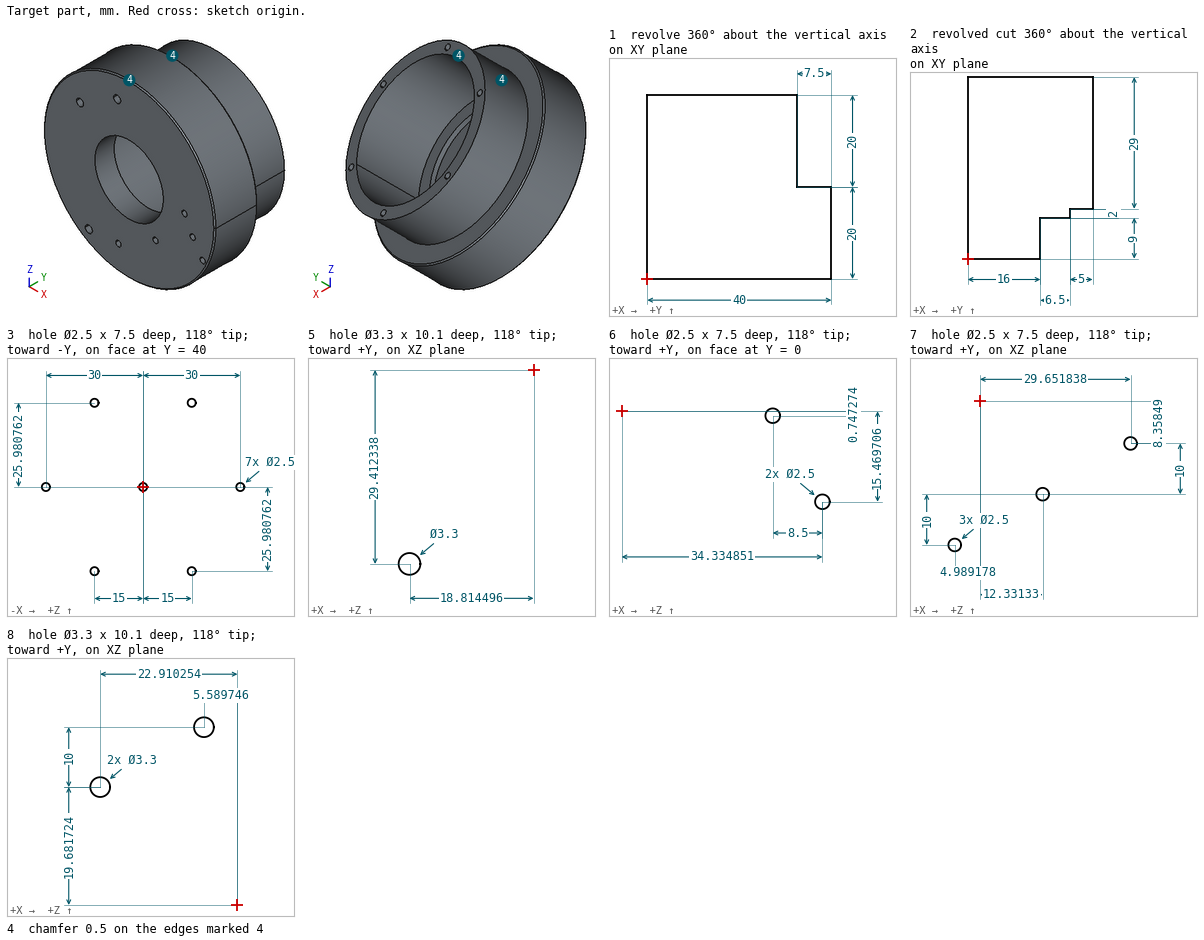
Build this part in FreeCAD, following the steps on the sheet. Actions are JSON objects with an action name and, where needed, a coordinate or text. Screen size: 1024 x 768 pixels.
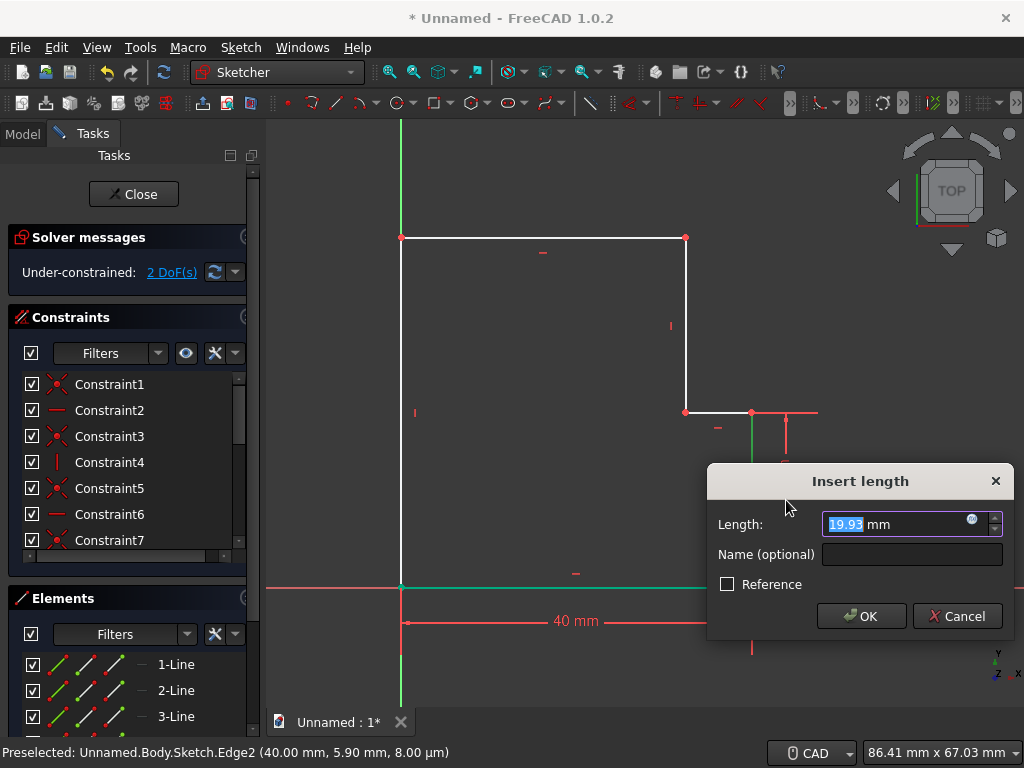
{"action": "type", "text": "20"}
{"action": "key", "text": "Return"}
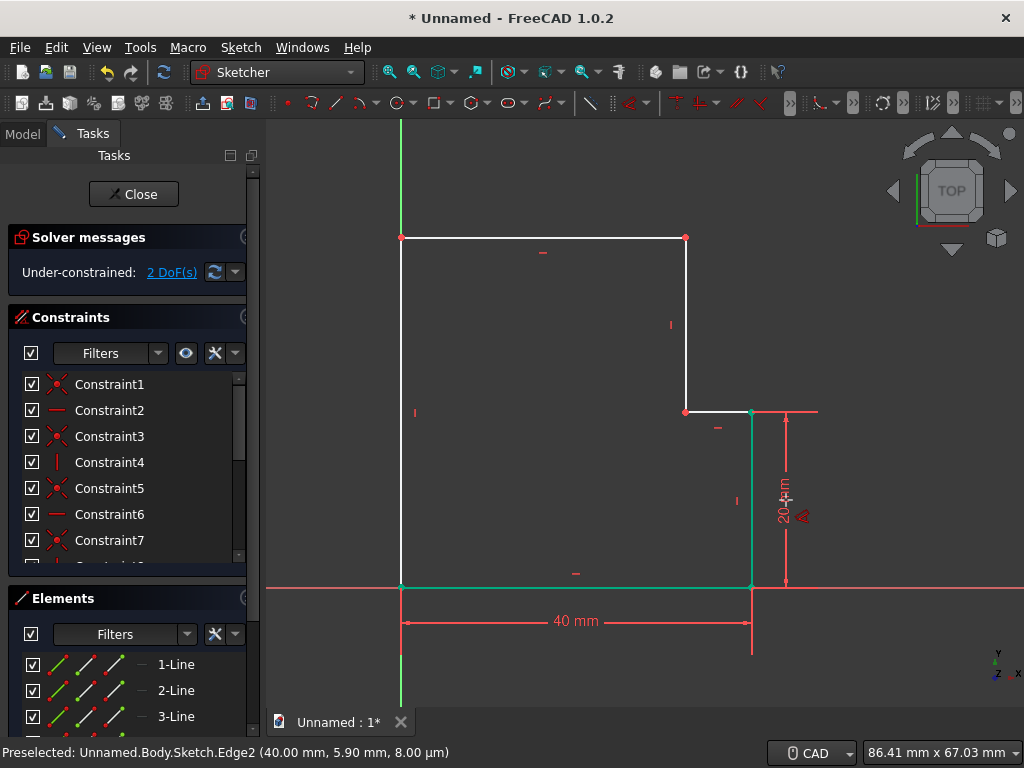
{"action": "left_click", "coordinate": [686, 360]}
{"action": "left_click", "coordinate": [720, 325]}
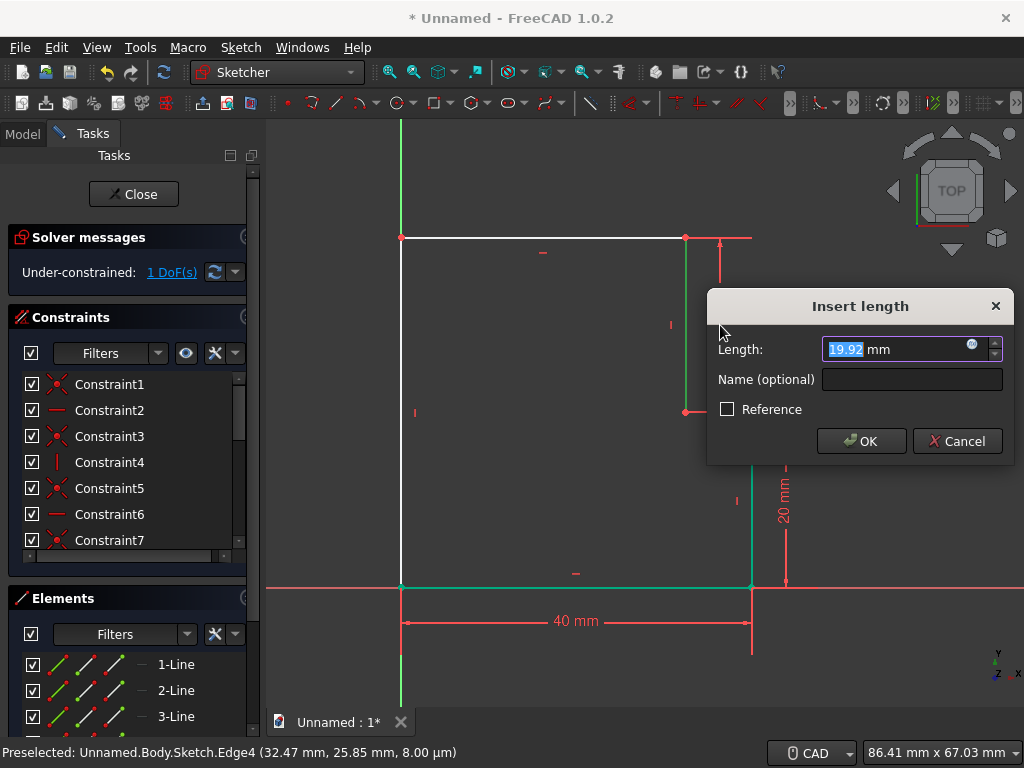
{"action": "type", "text": "20"}
{"action": "key", "text": "Return"}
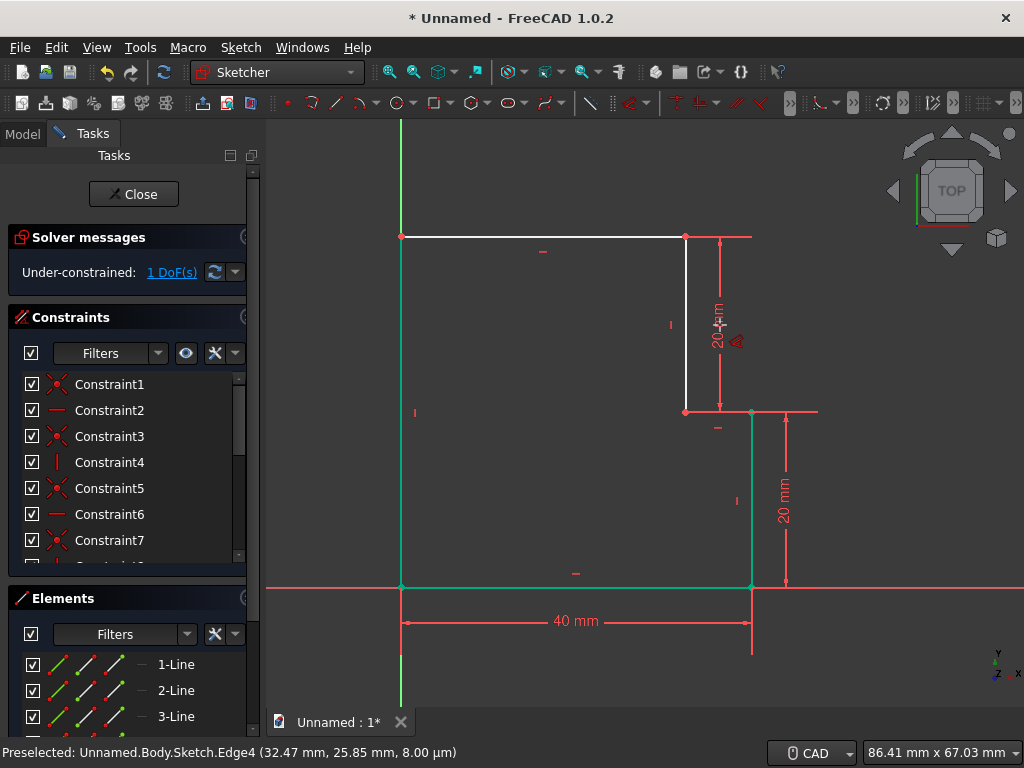
{"action": "left_click", "coordinate": [732, 412]}
{"action": "left_click", "coordinate": [719, 446]}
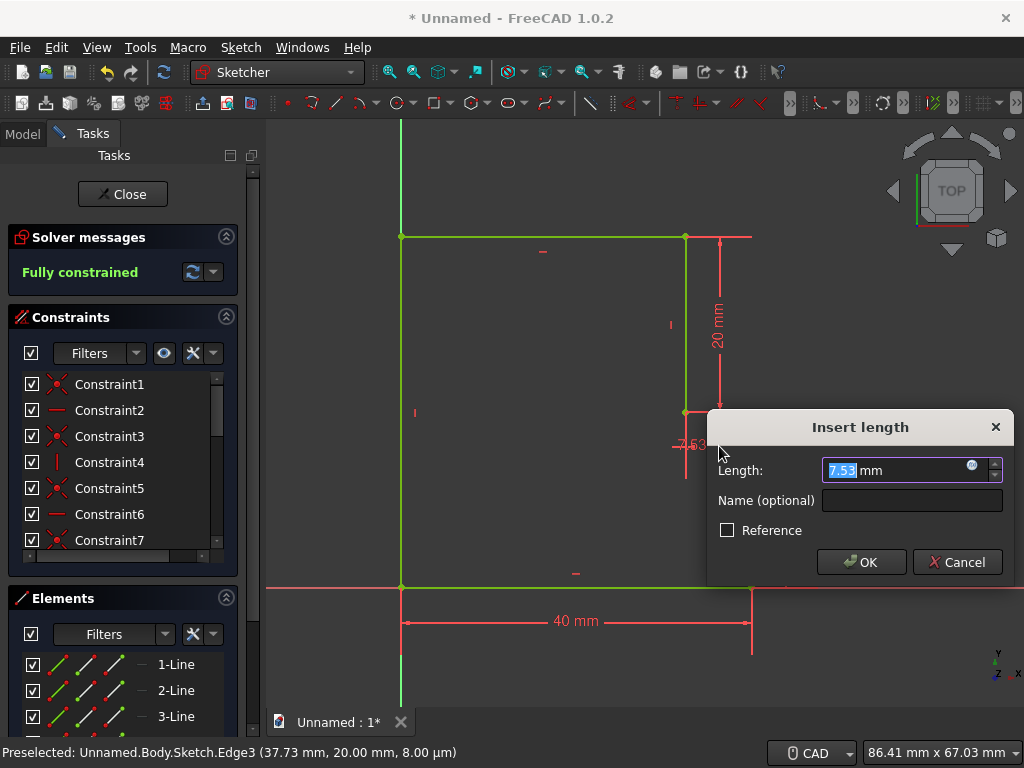
{"action": "type", "text": "7.5"}
{"action": "key", "text": "Return"}
{"action": "key", "text": "Escape"}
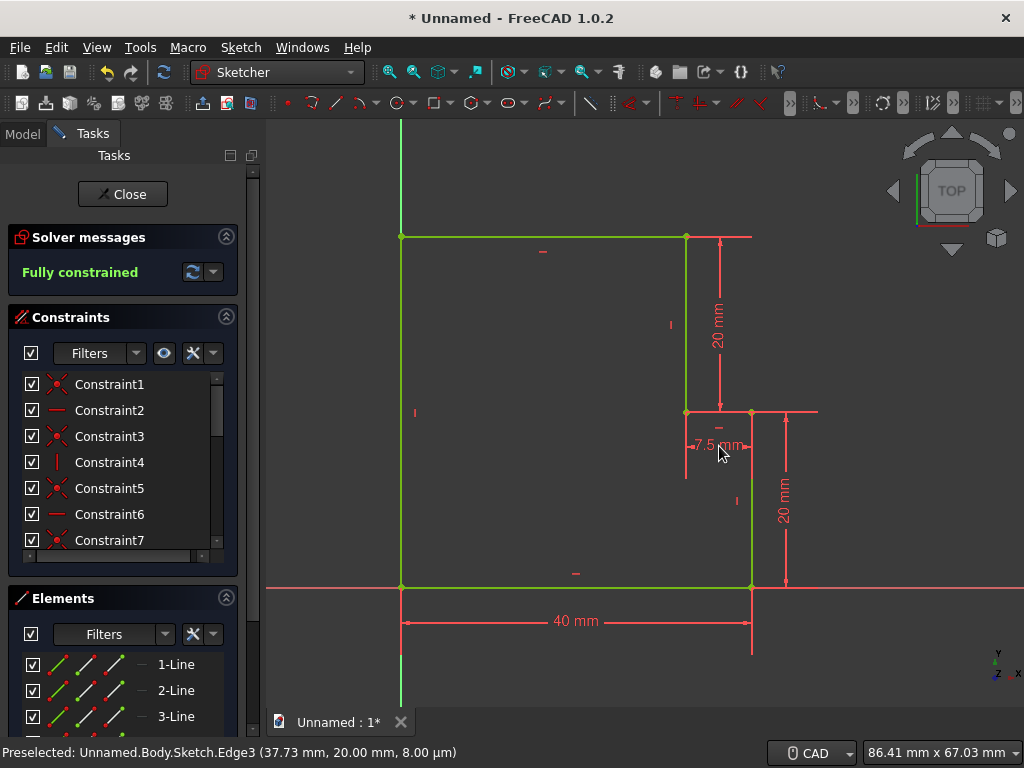
{"action": "left_click", "coordinate": [123, 194]}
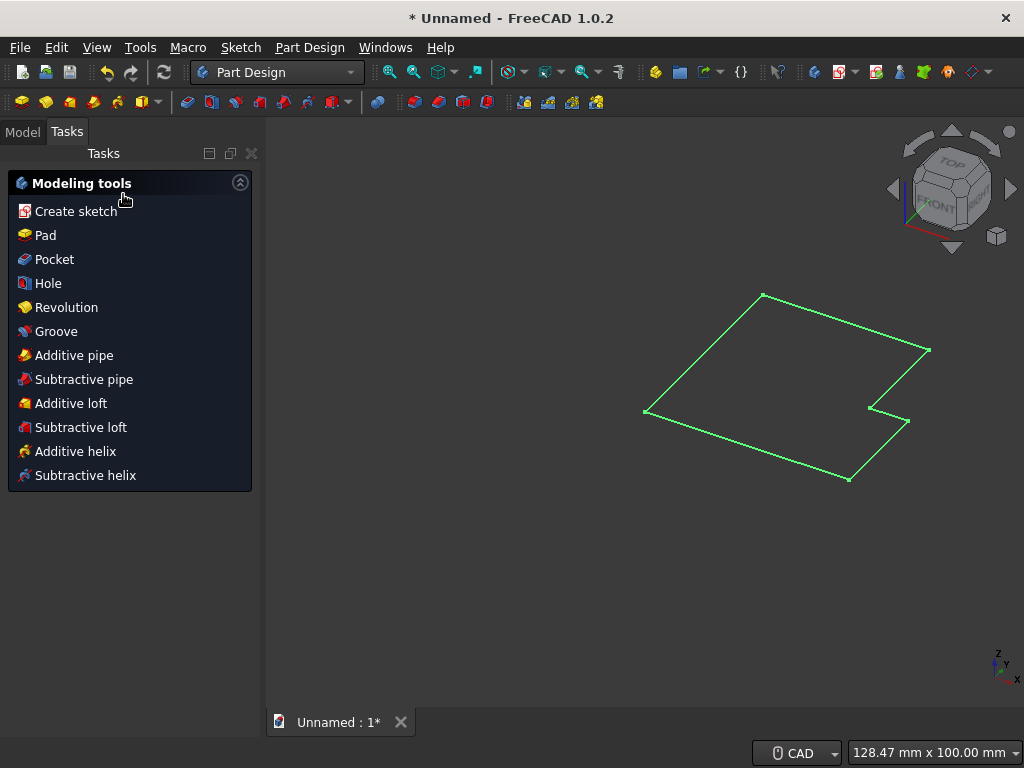
{"action": "left_click", "coordinate": [46, 102]}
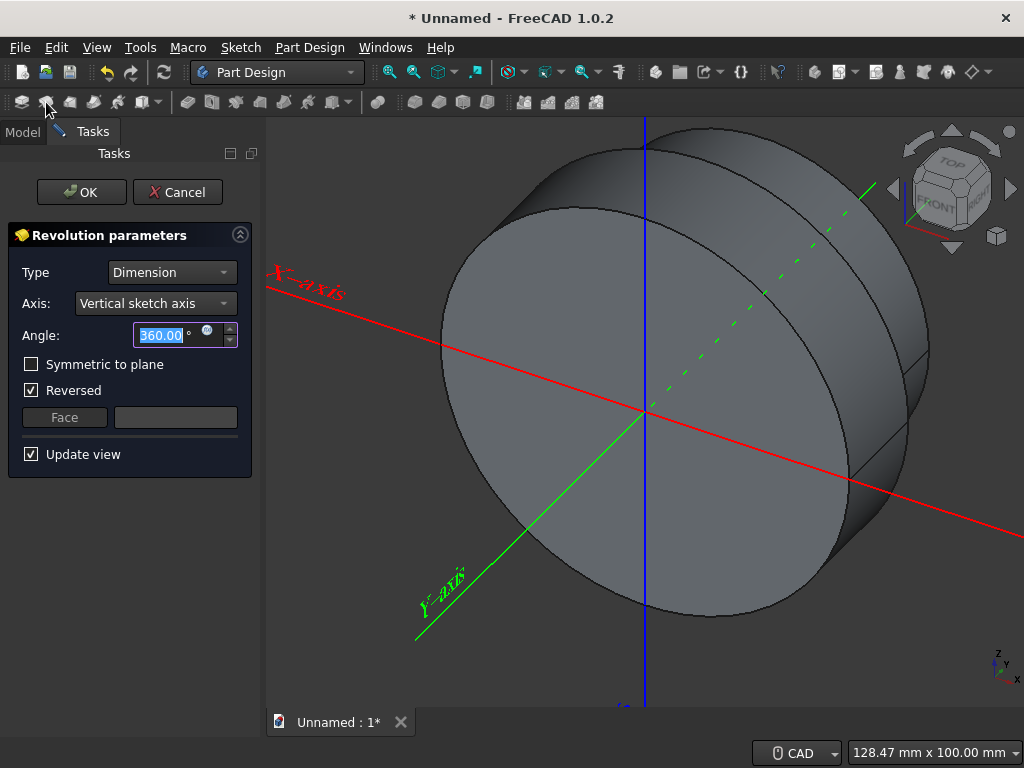
{"action": "left_click", "coordinate": [82, 192]}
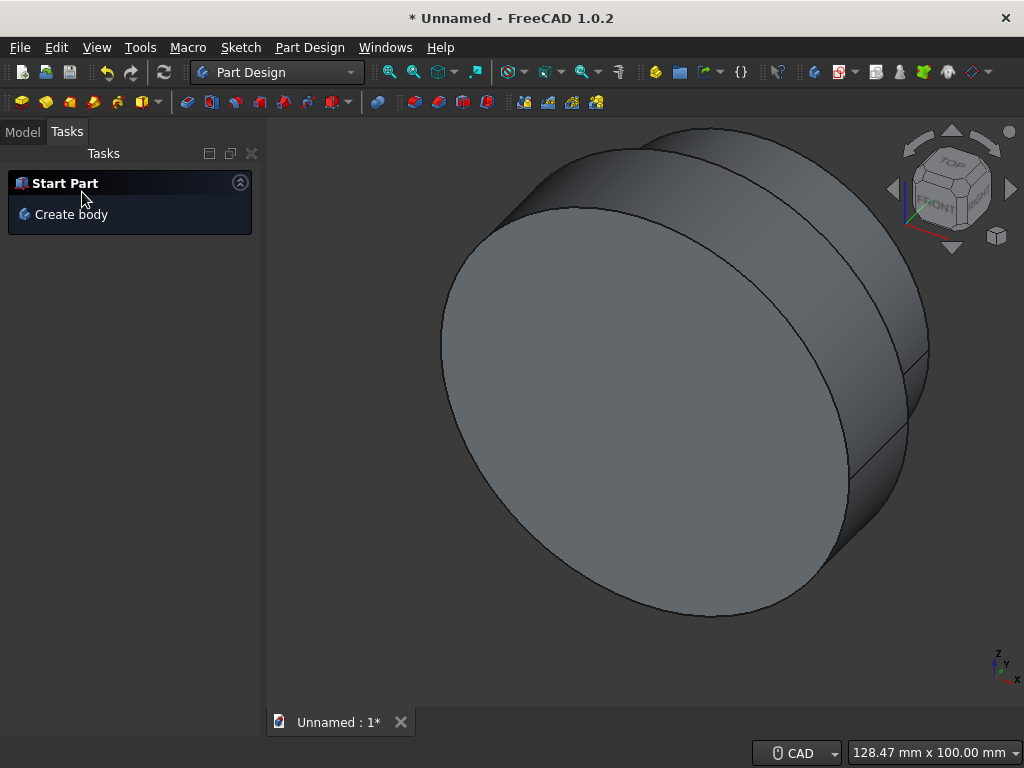
{"action": "left_click", "coordinate": [390, 72]}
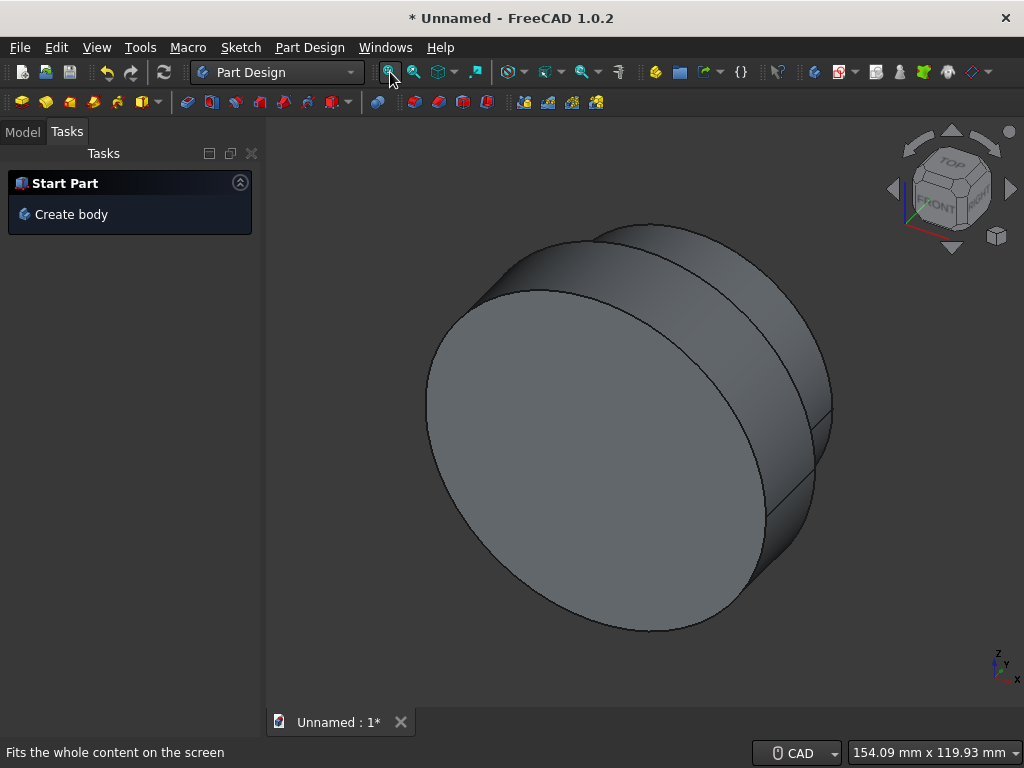
{"action": "left_click", "coordinate": [840, 72]}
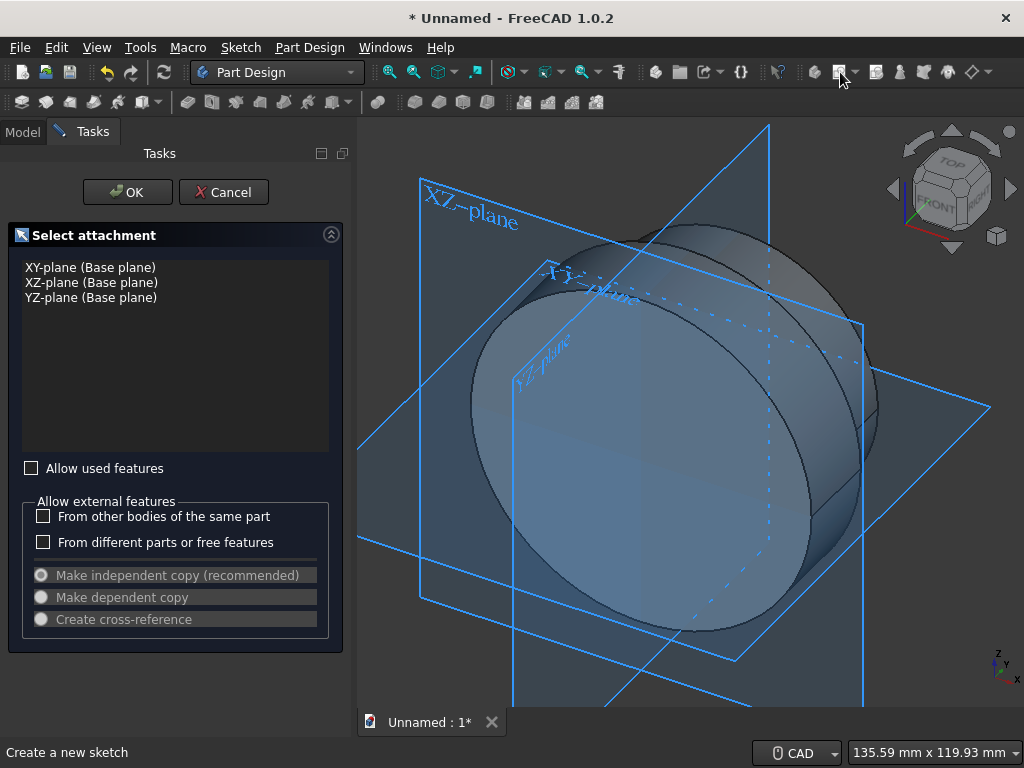
{"action": "left_click", "coordinate": [82, 268]}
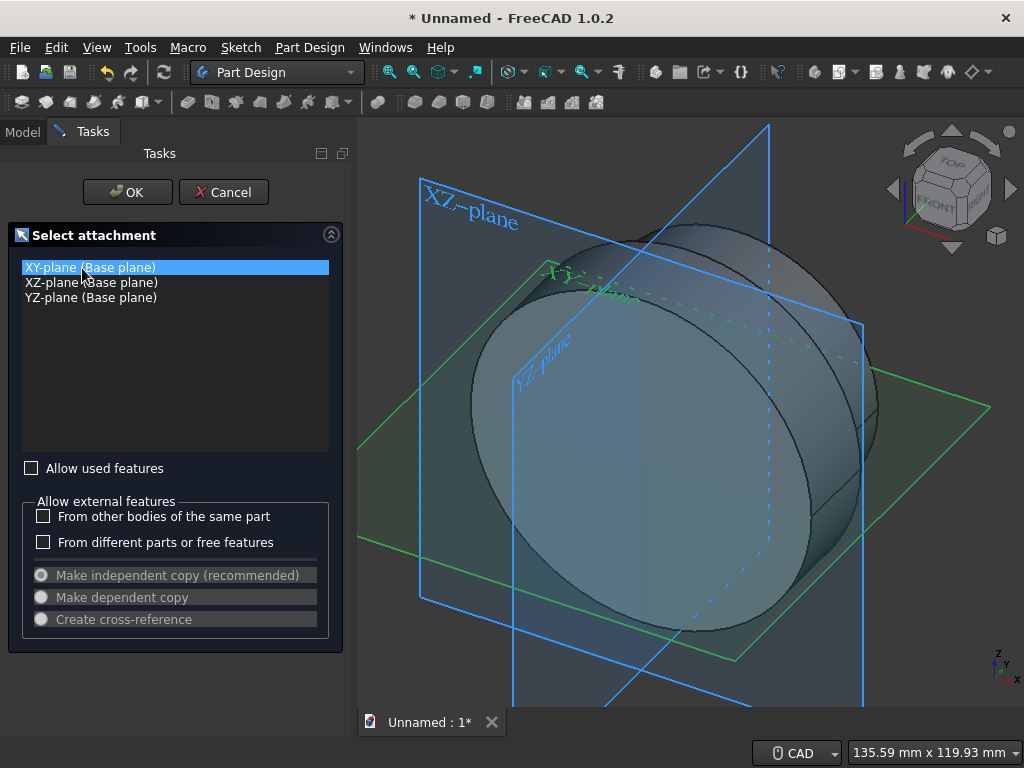
{"action": "left_click", "coordinate": [128, 192]}